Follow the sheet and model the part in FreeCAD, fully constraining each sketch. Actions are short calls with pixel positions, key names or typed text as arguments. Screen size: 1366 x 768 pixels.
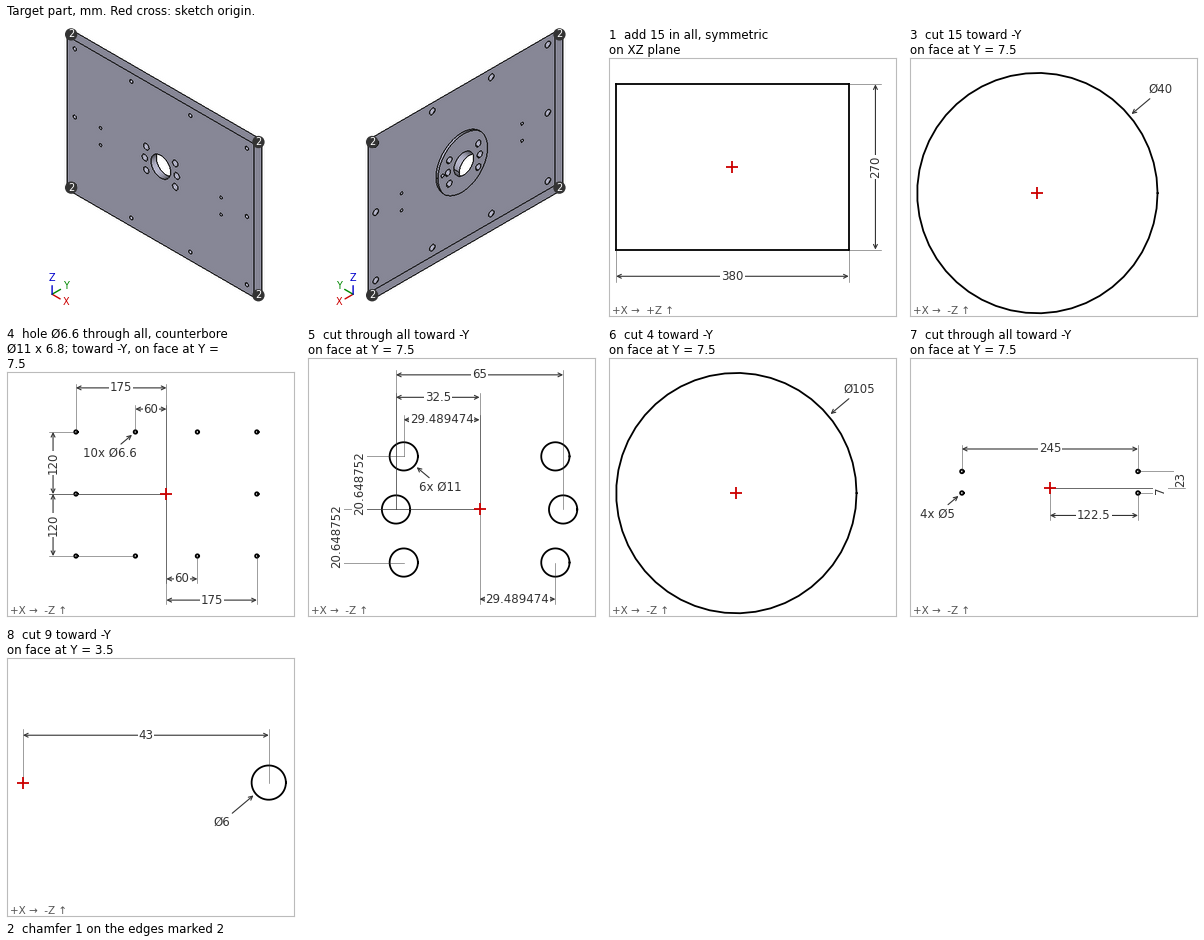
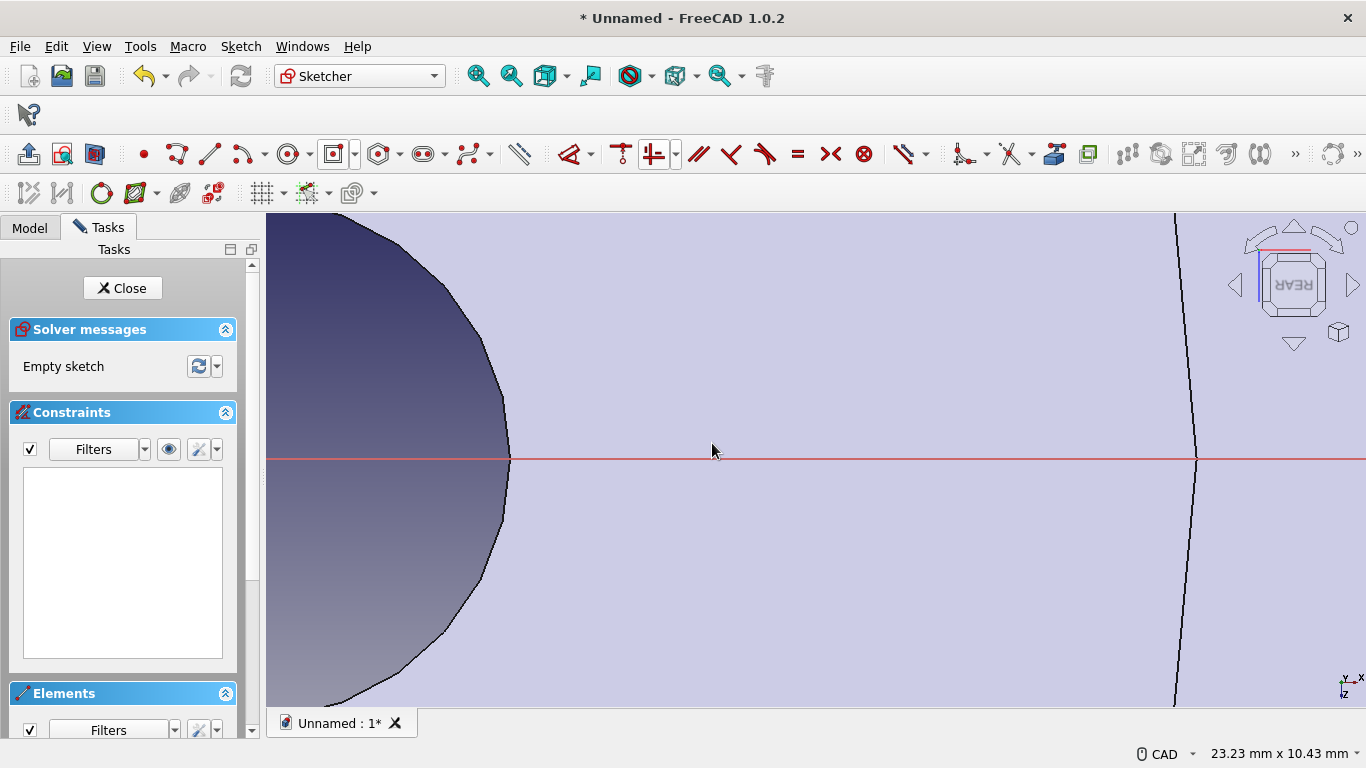
click(288, 154)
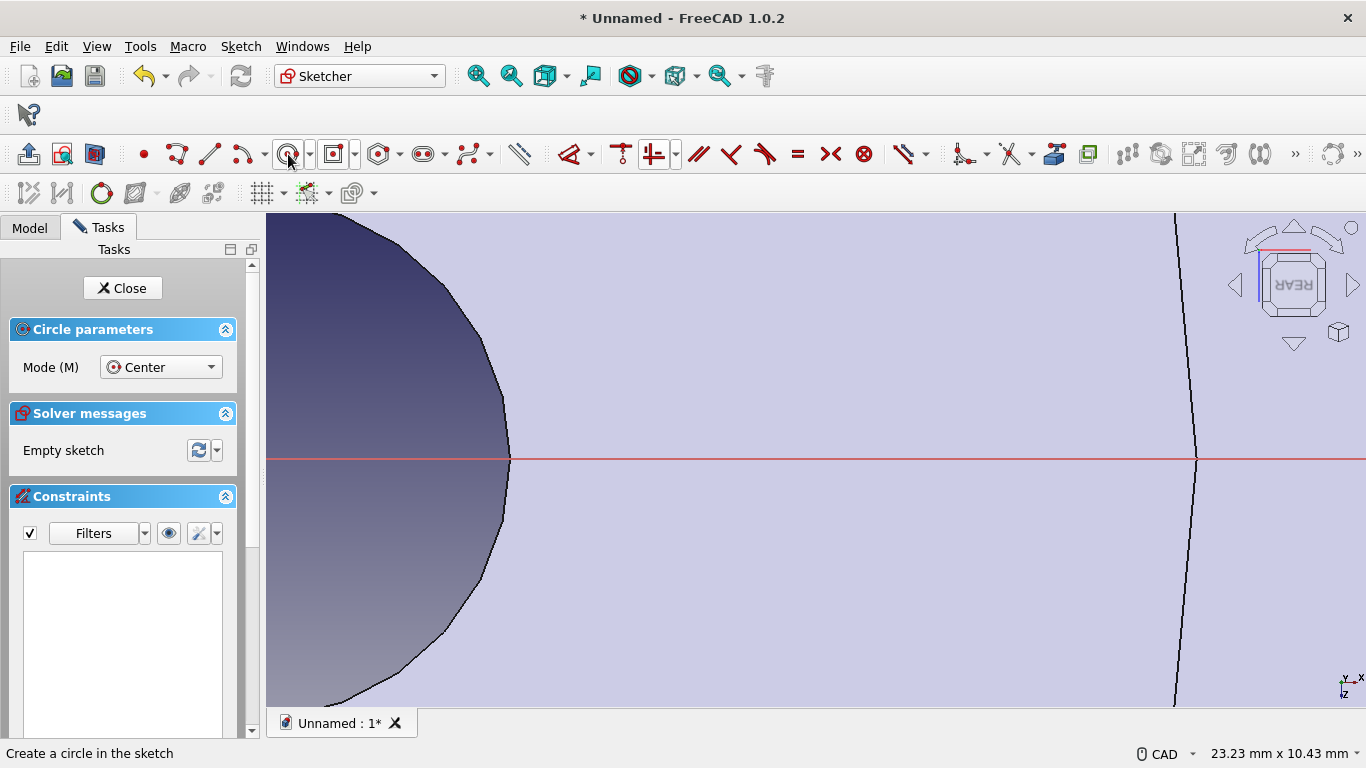
click(747, 459)
click(847, 359)
key(Escape)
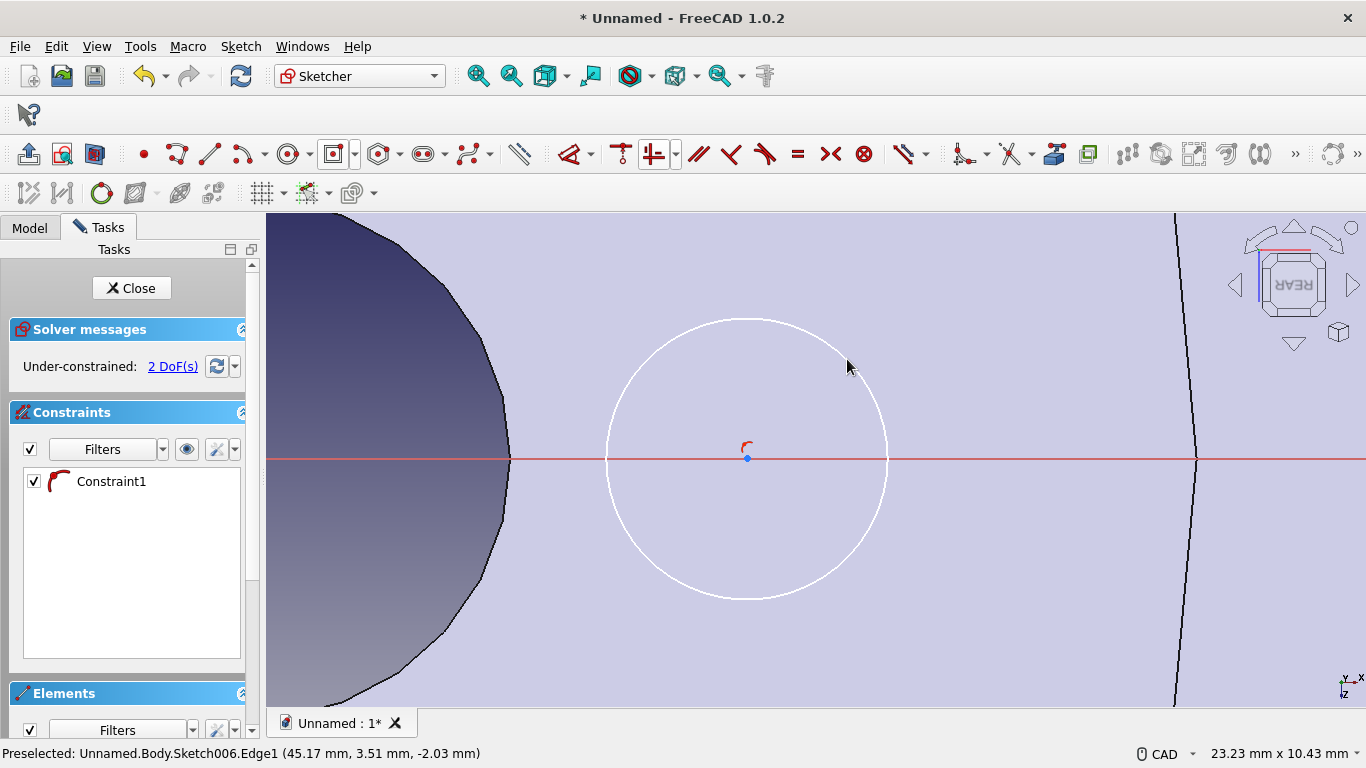
click(568, 154)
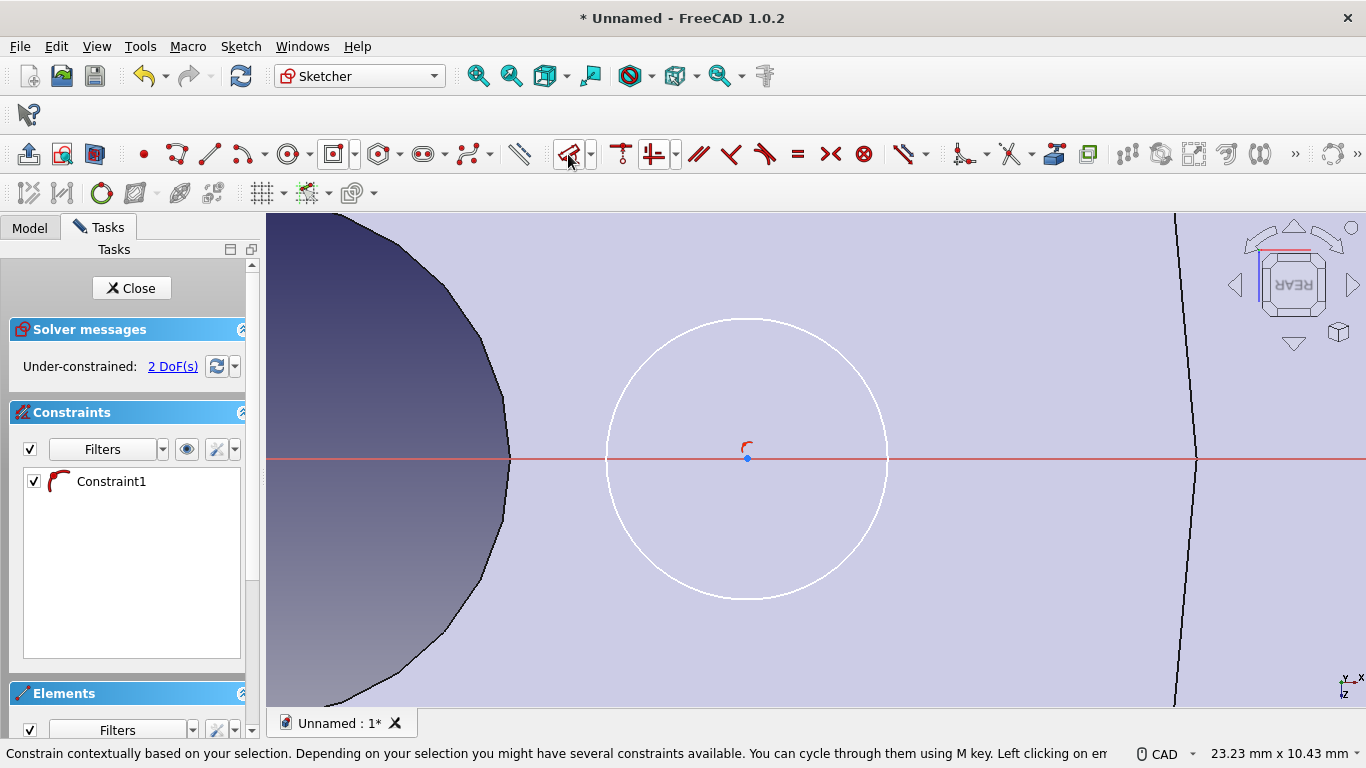
click(846, 359)
click(869, 336)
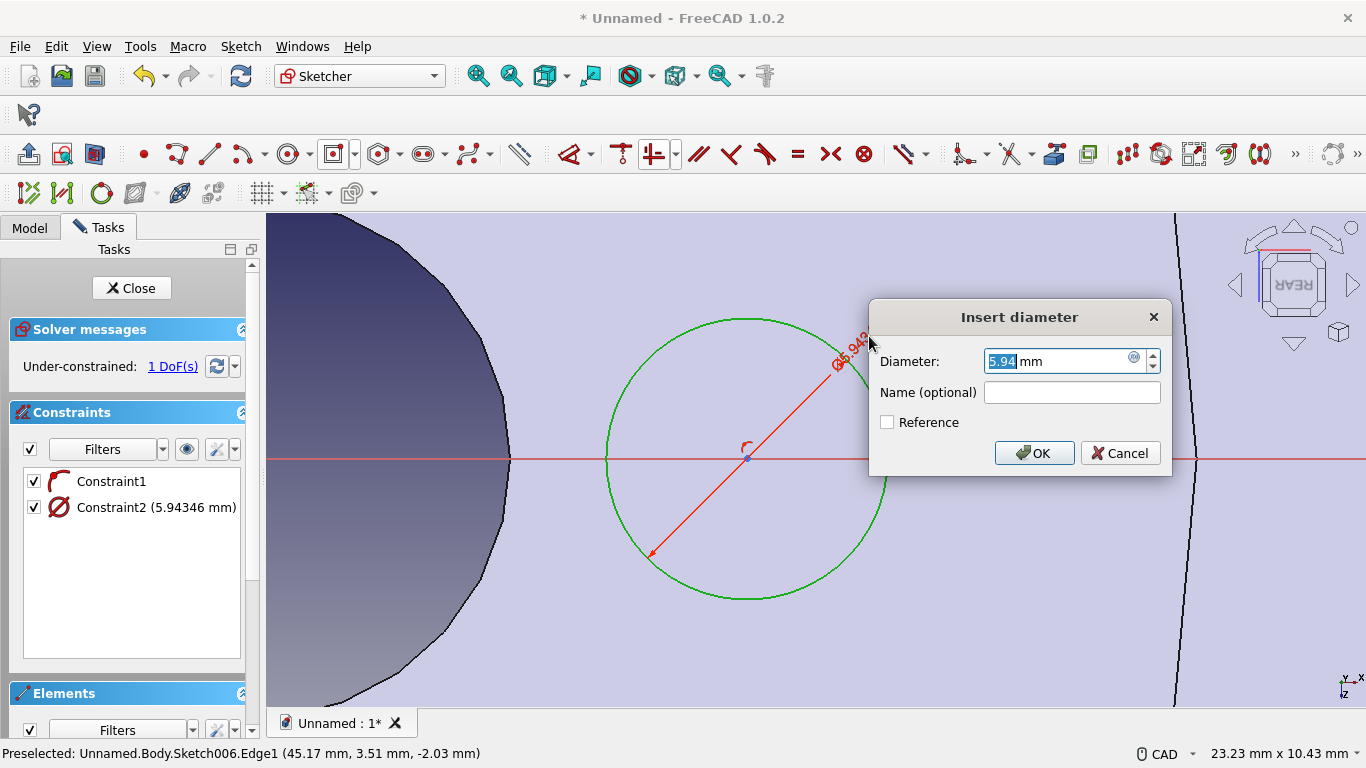
text(6)
key(Return)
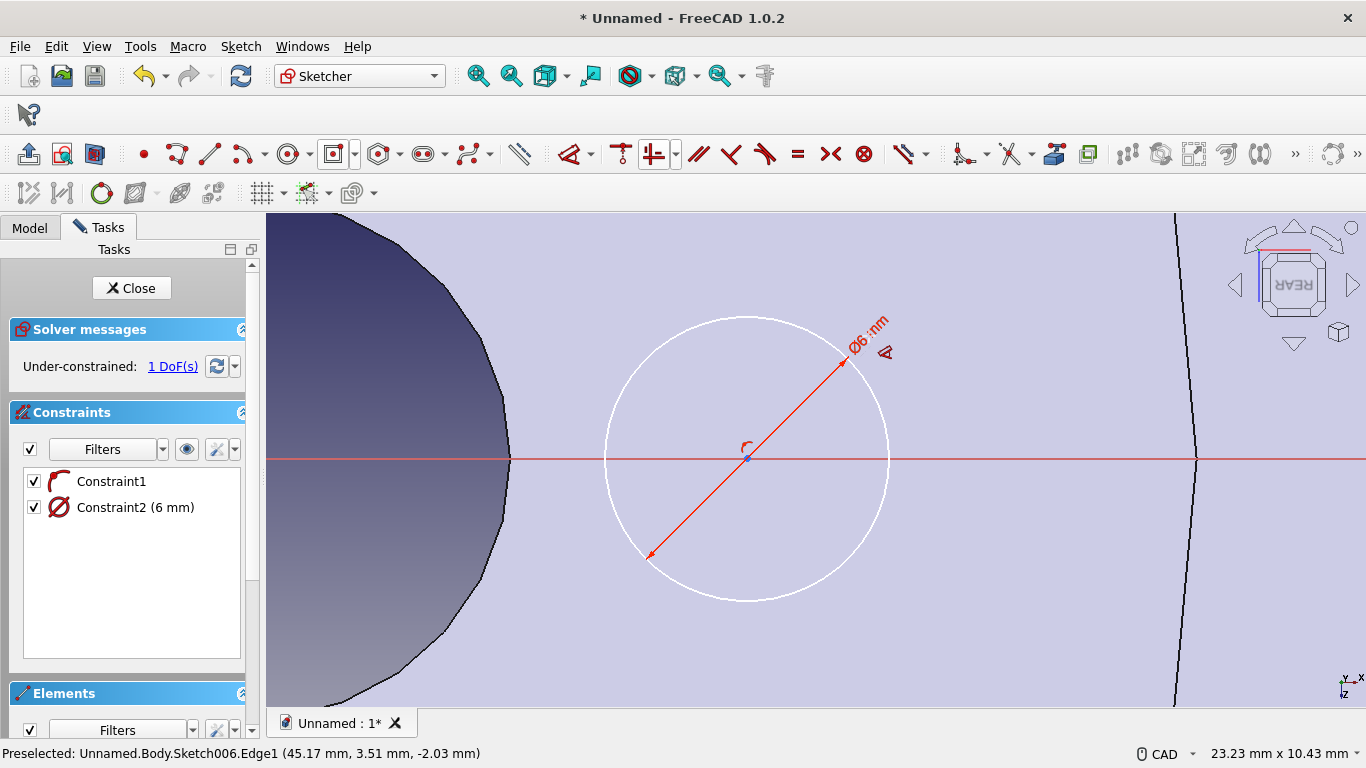
click(747, 459)
click(521, 493)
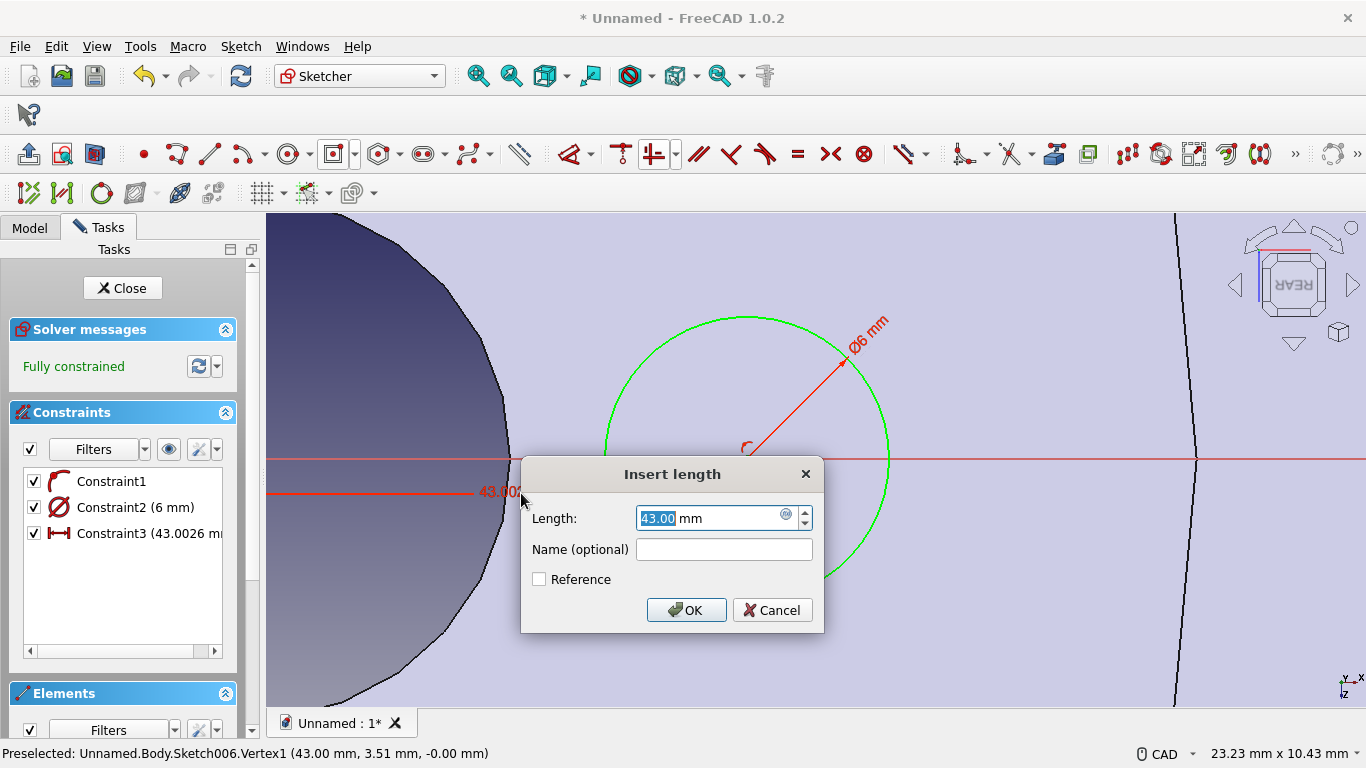
text(43)
key(Return)
key(Escape)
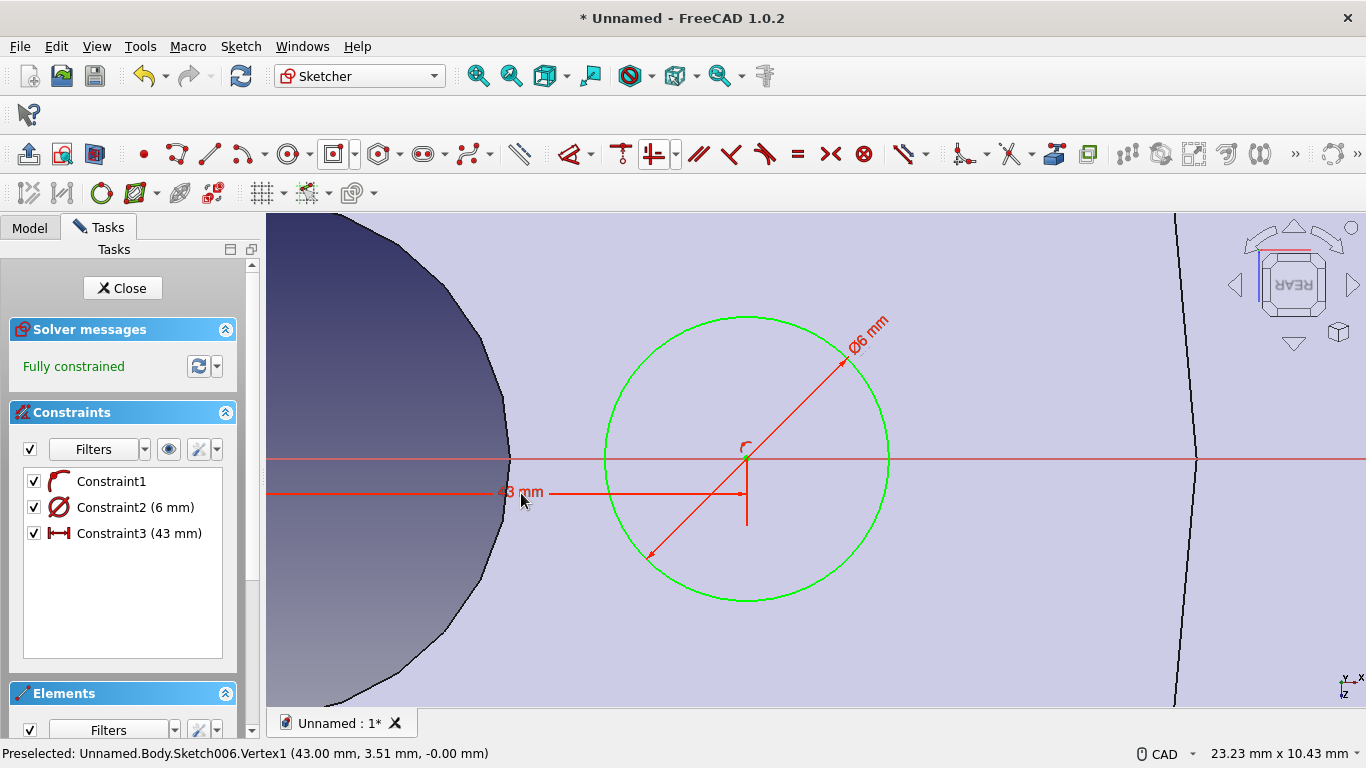
click(123, 288)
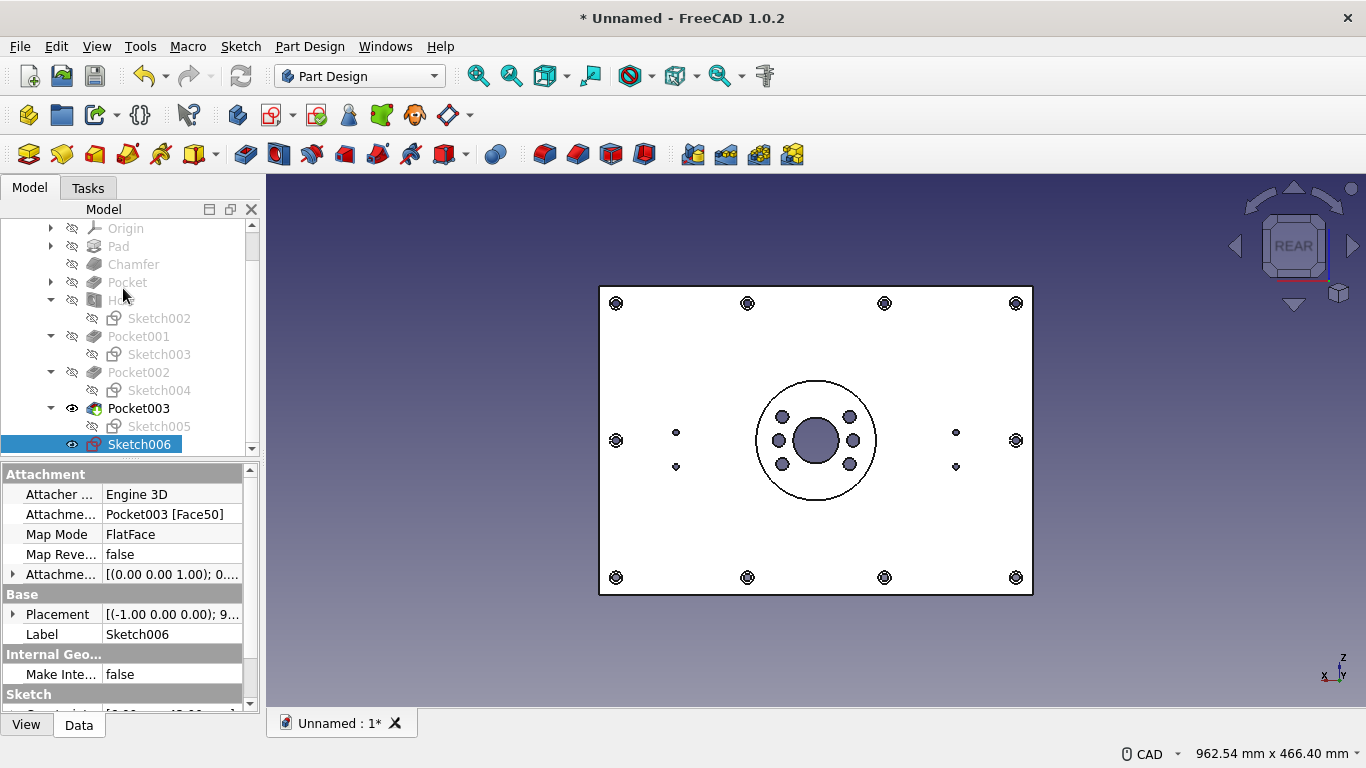
click(246, 154)